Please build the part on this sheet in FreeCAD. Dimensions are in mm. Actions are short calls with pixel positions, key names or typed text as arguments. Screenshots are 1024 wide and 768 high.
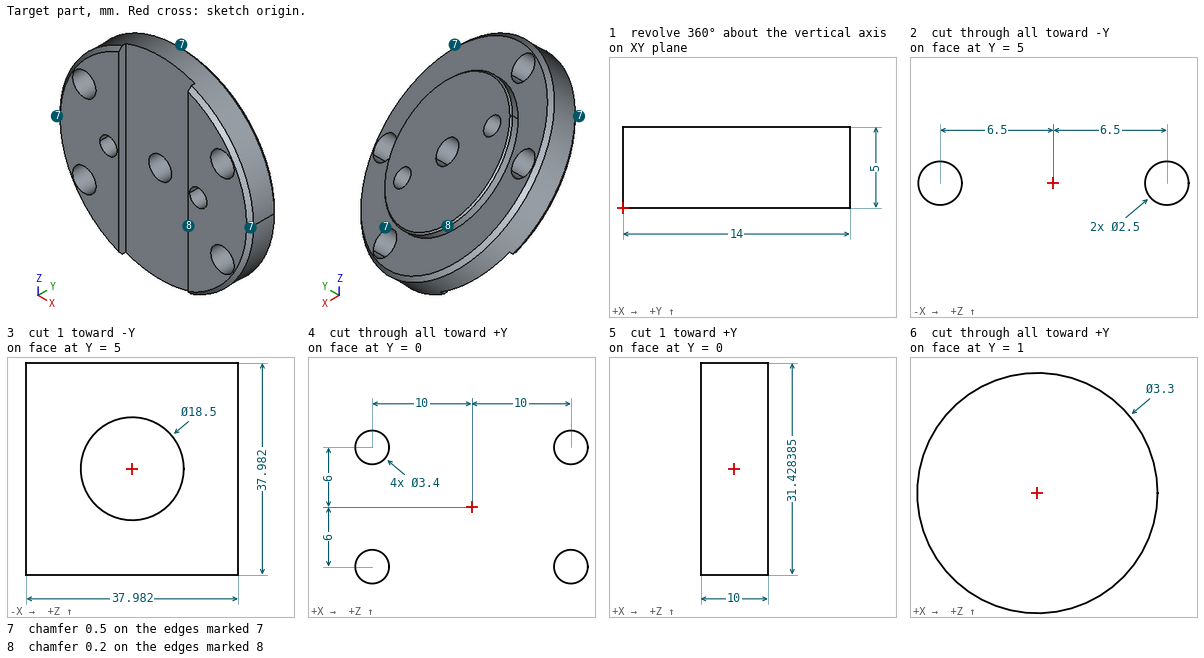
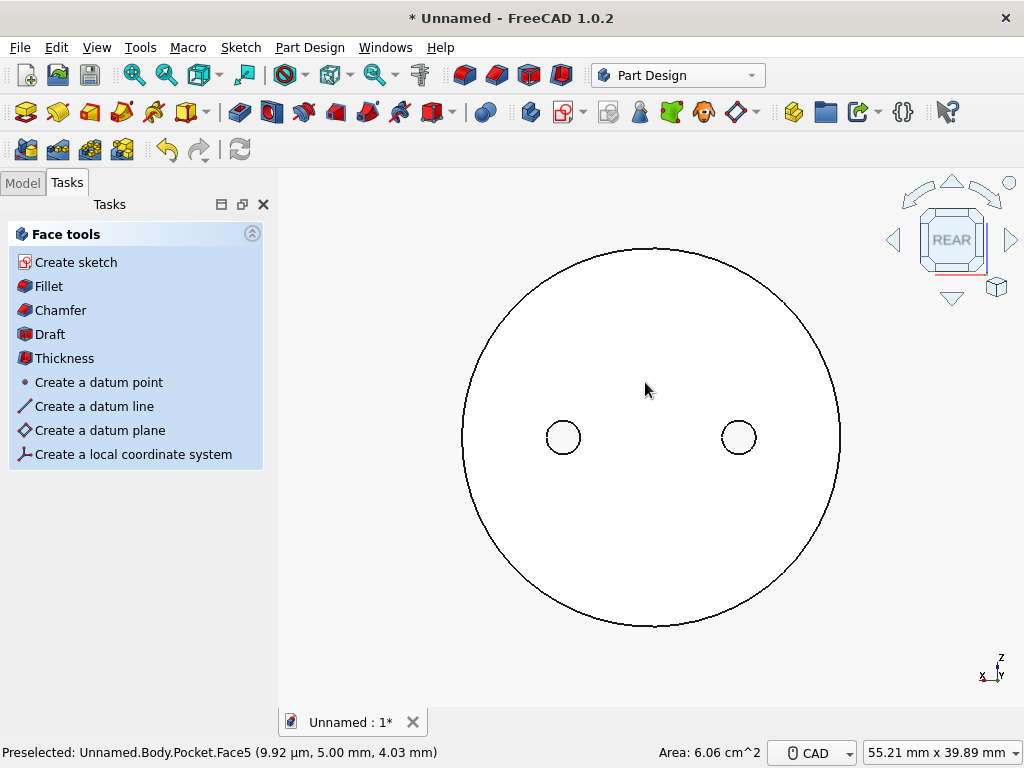
click(564, 112)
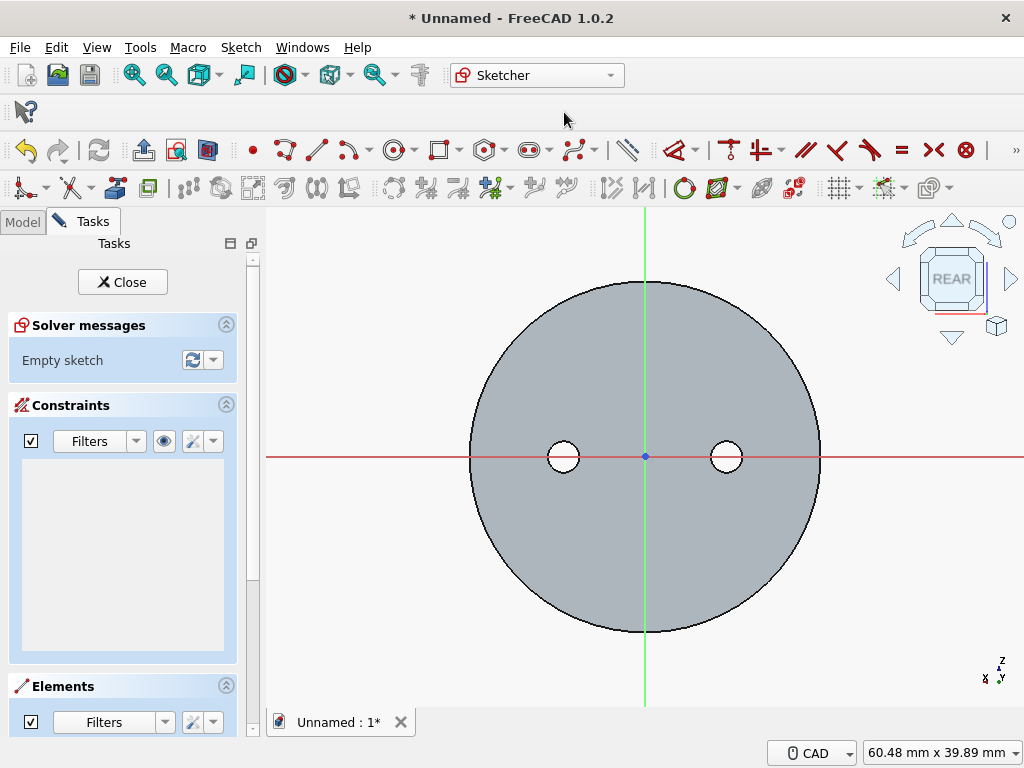
scroll(437, 457, down, 2)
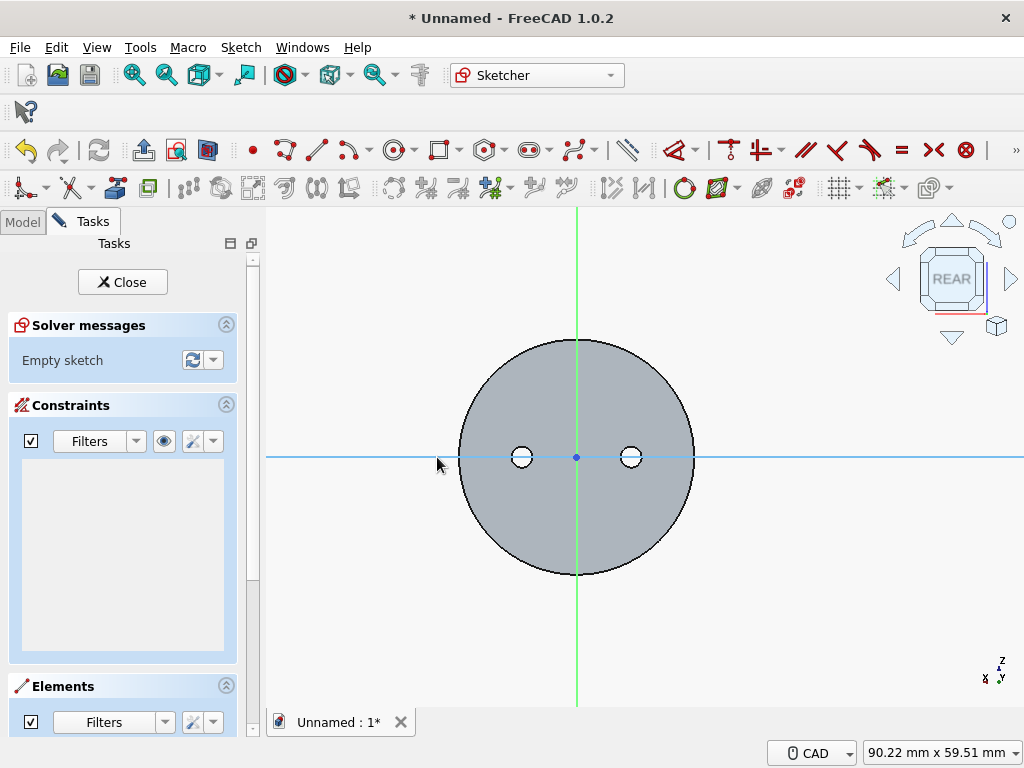
key(g)
key(v)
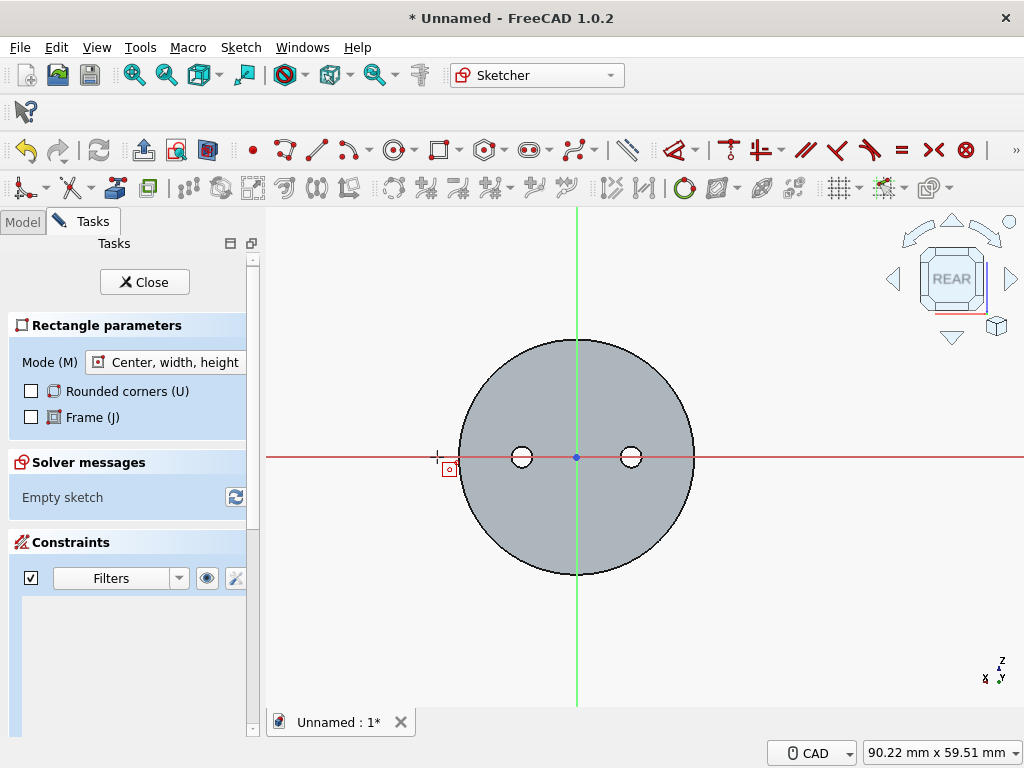
click(577, 457)
click(736, 298)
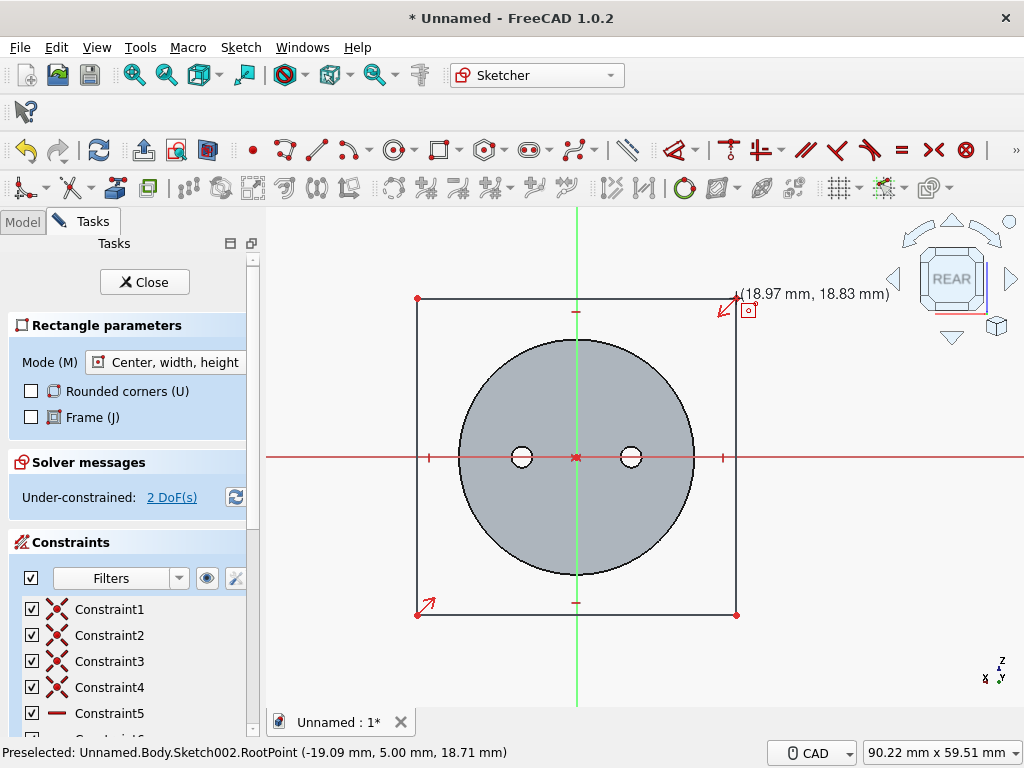
click(394, 150)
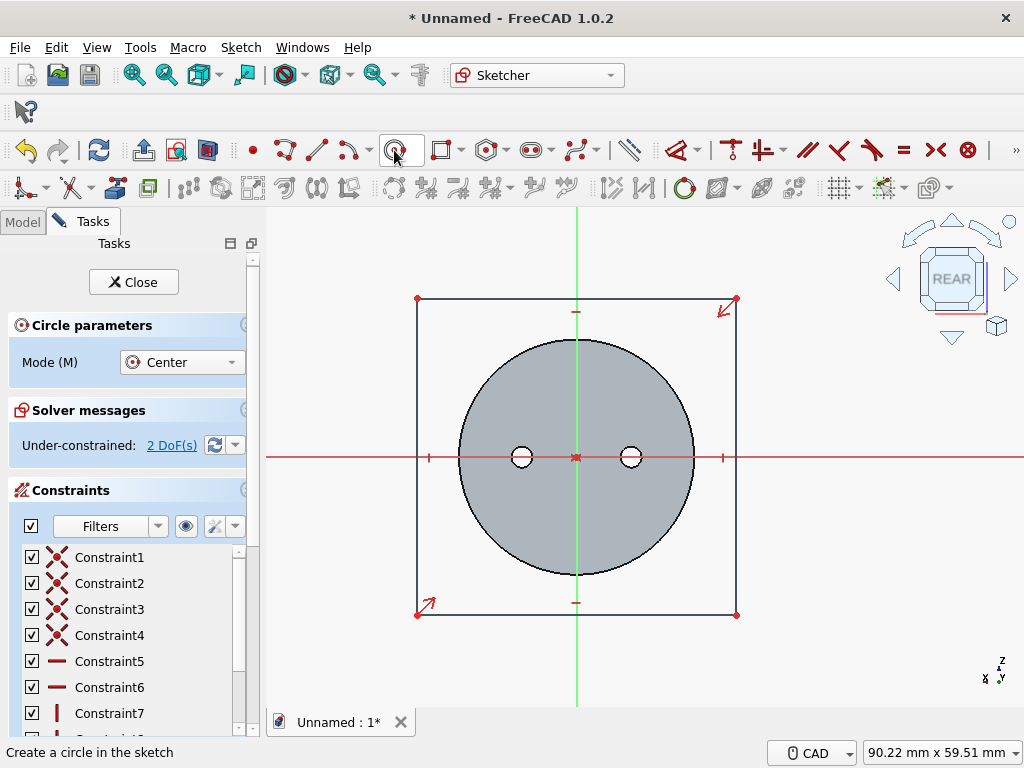
click(577, 457)
click(632, 402)
key(Escape)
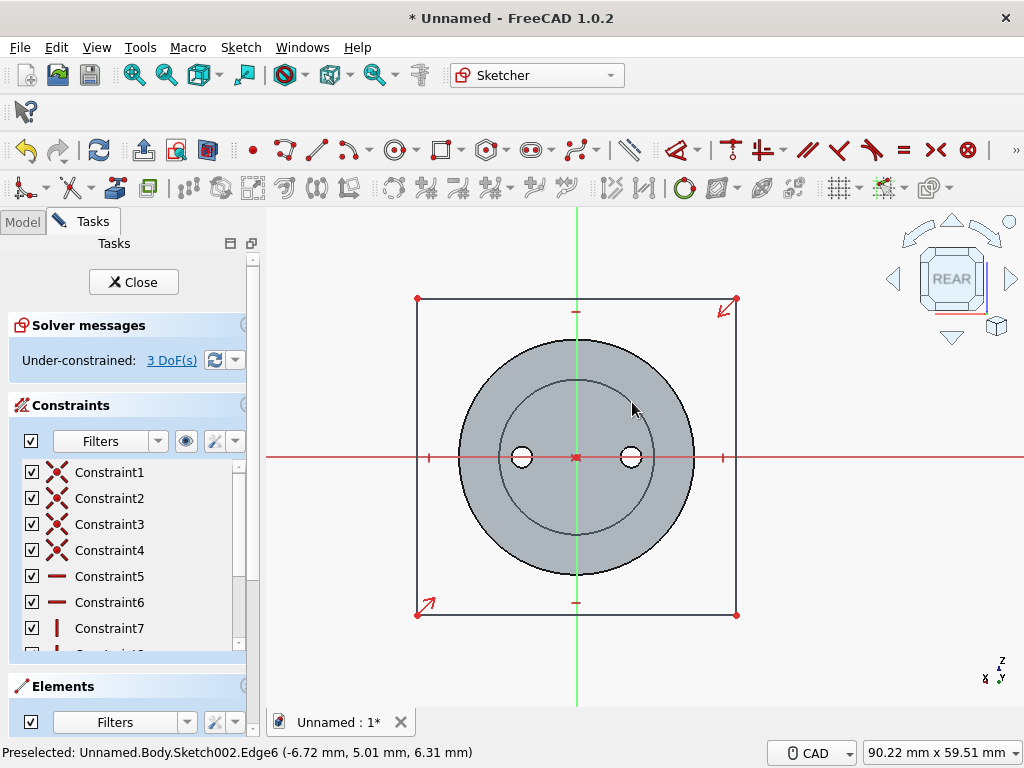
key(d)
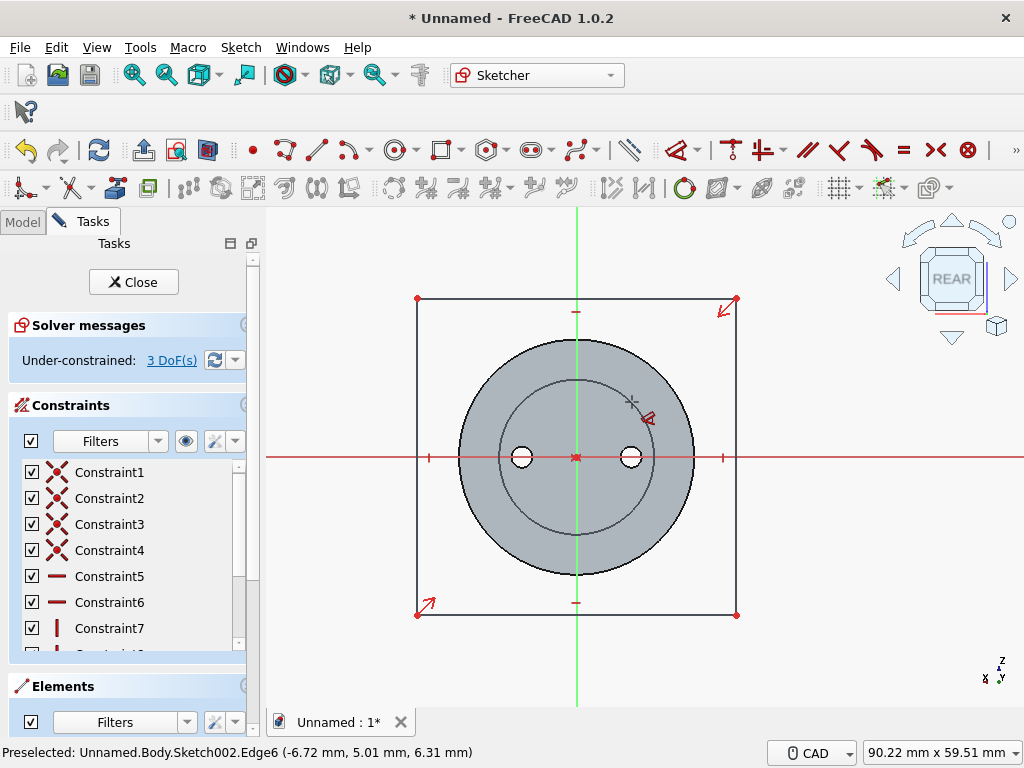
click(631, 402)
click(653, 379)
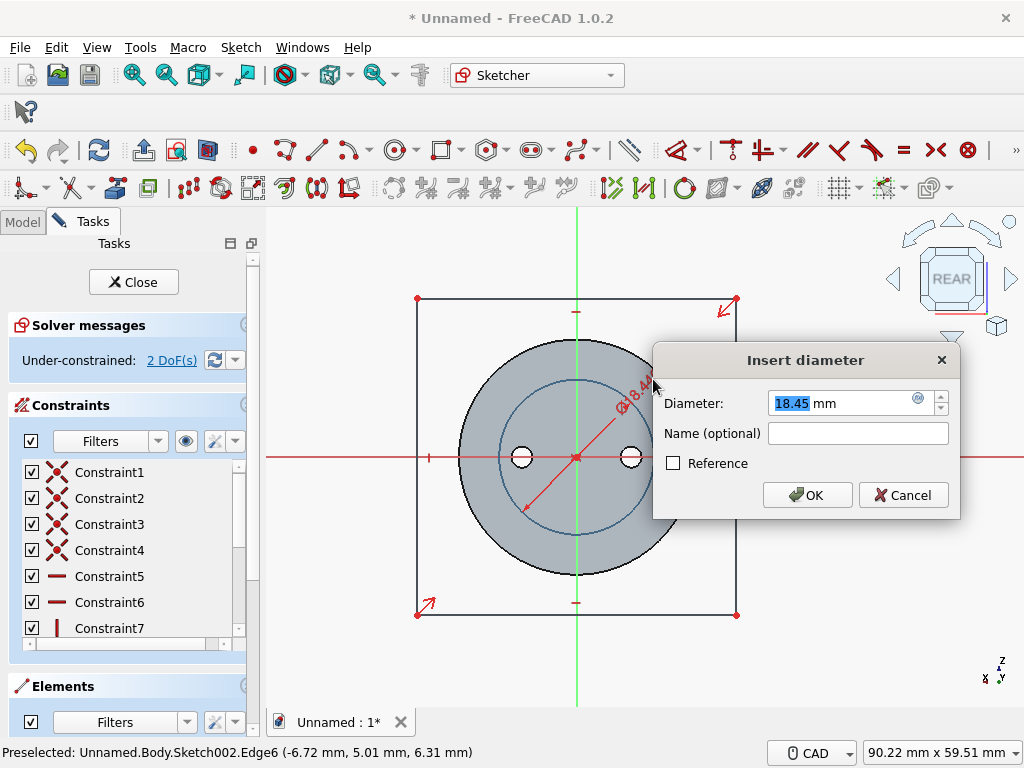
text(18.5)
key(Return)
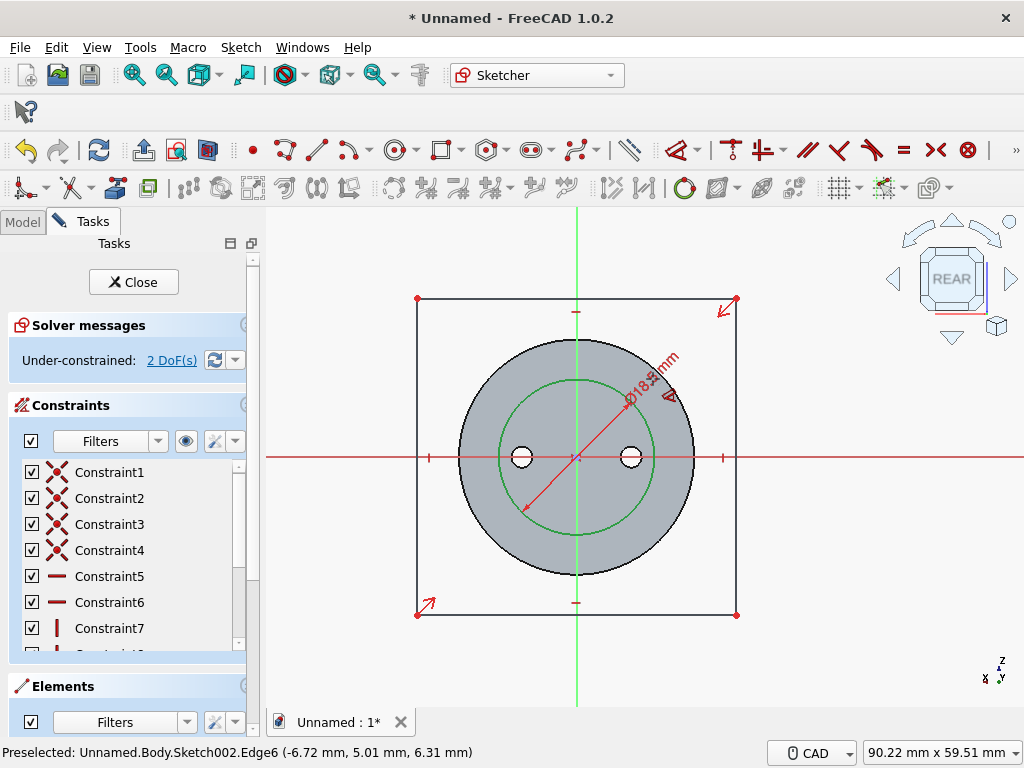
click(513, 615)
click(503, 649)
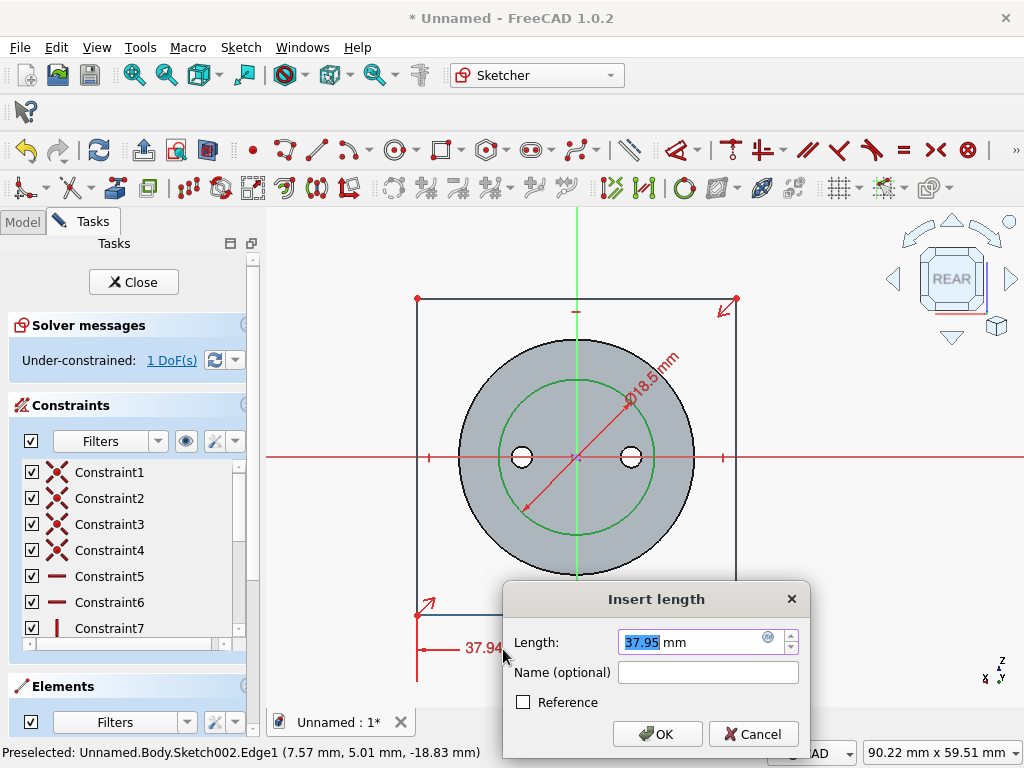
text(37.982)
key(Return)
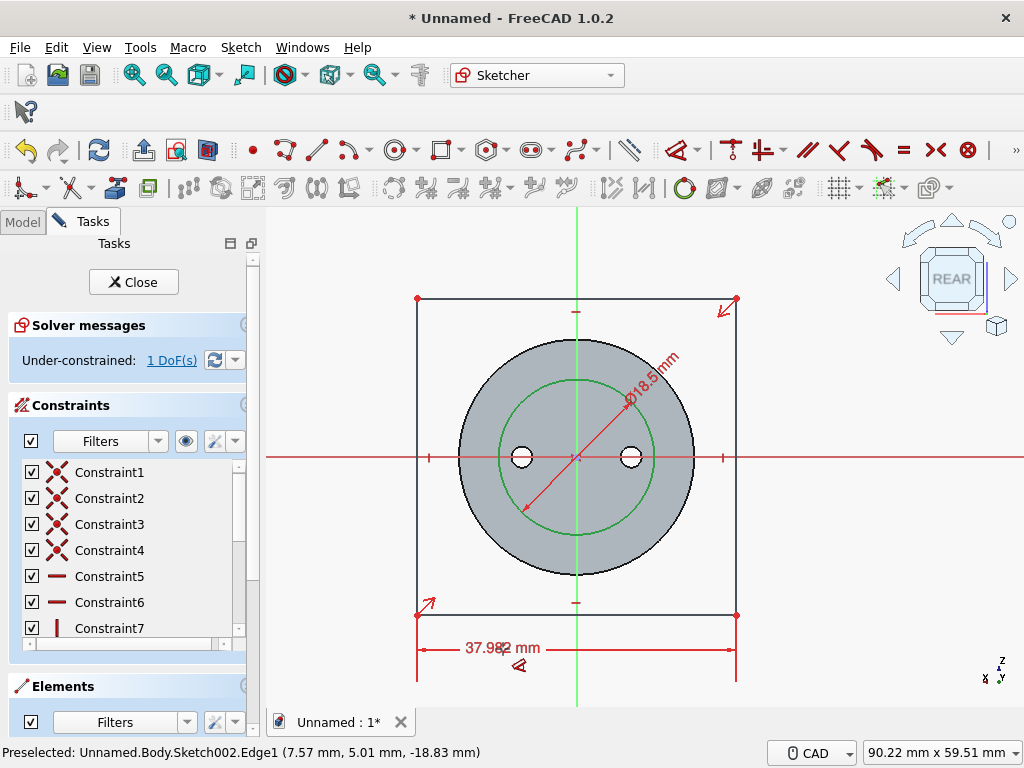
click(736, 520)
click(770, 384)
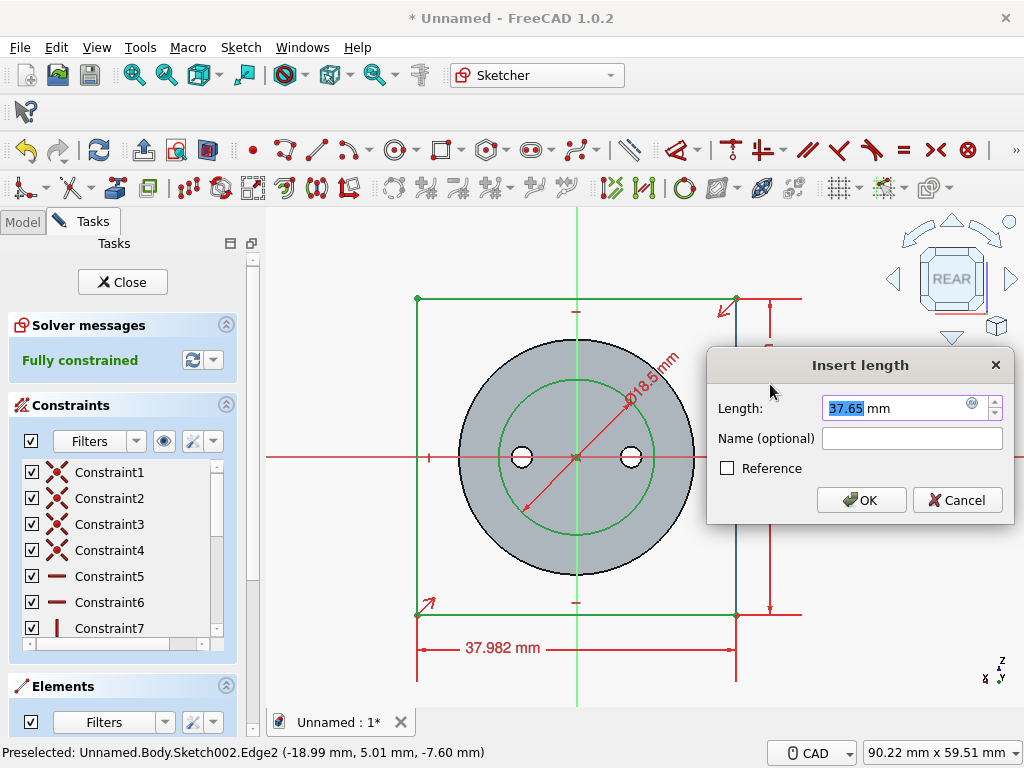
text(37.982)
key(Return)
key(Escape)